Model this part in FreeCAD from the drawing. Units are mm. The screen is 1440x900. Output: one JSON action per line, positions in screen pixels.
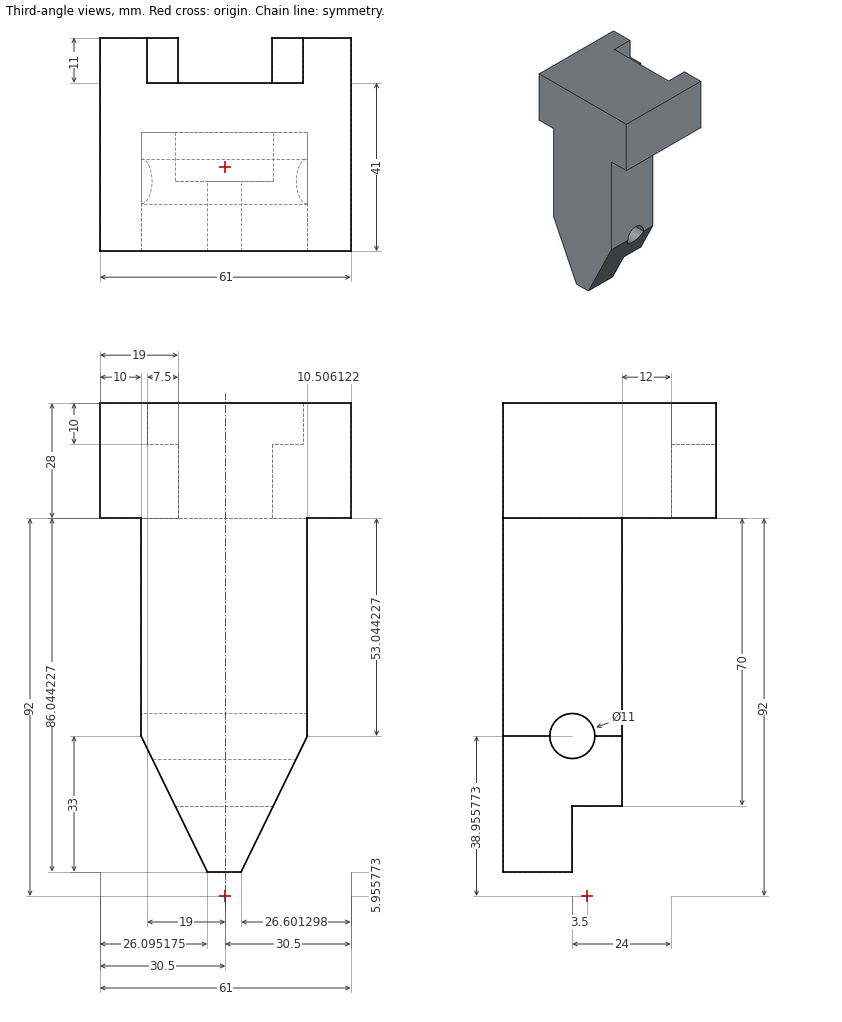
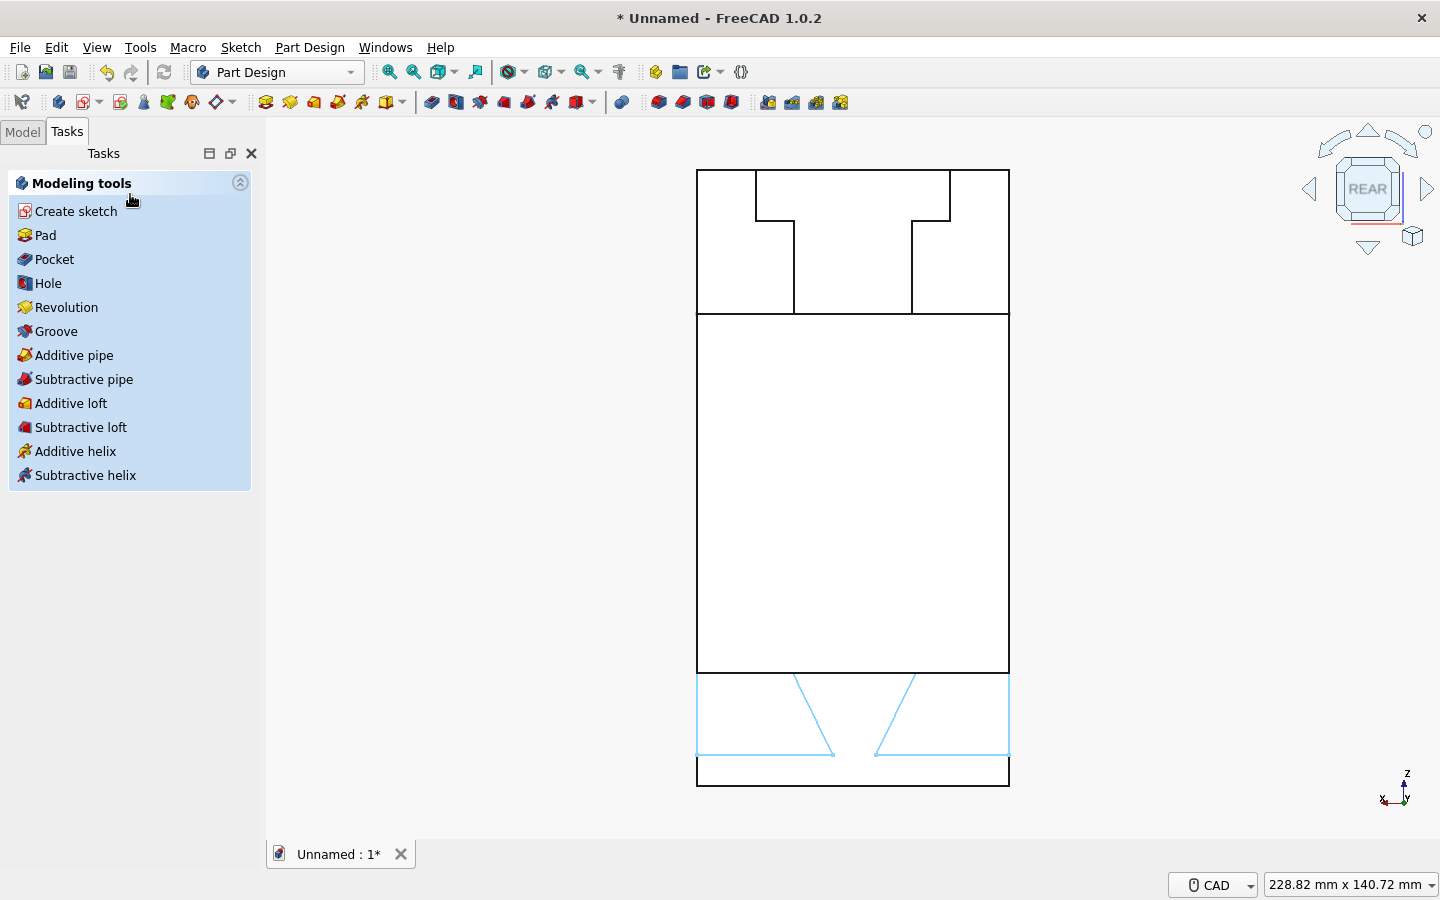
{"action": "left_click", "coordinate": [432, 102]}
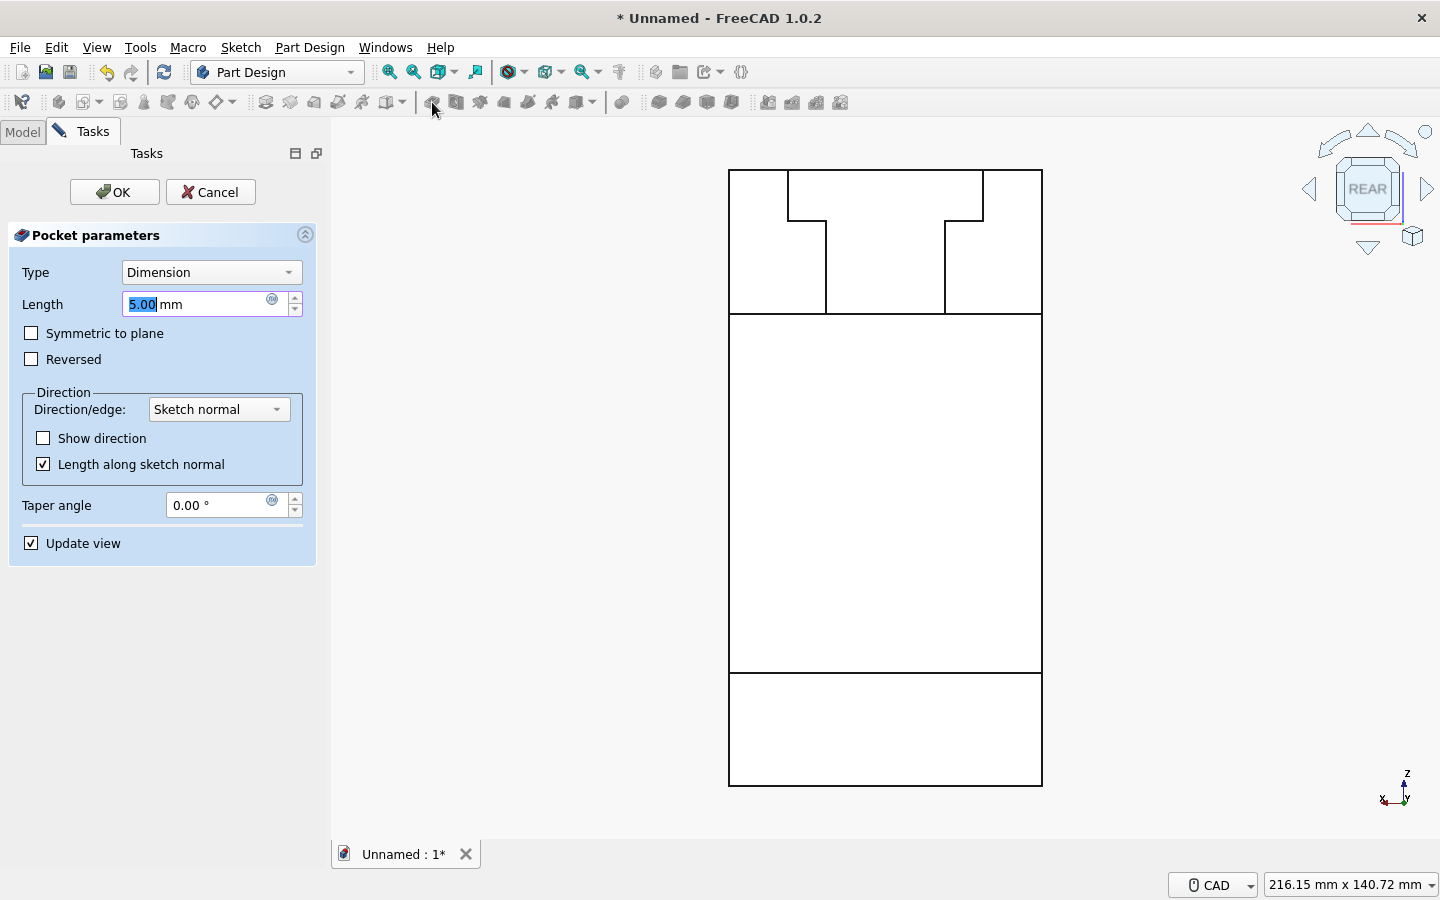
{"action": "left_click", "coordinate": [212, 272]}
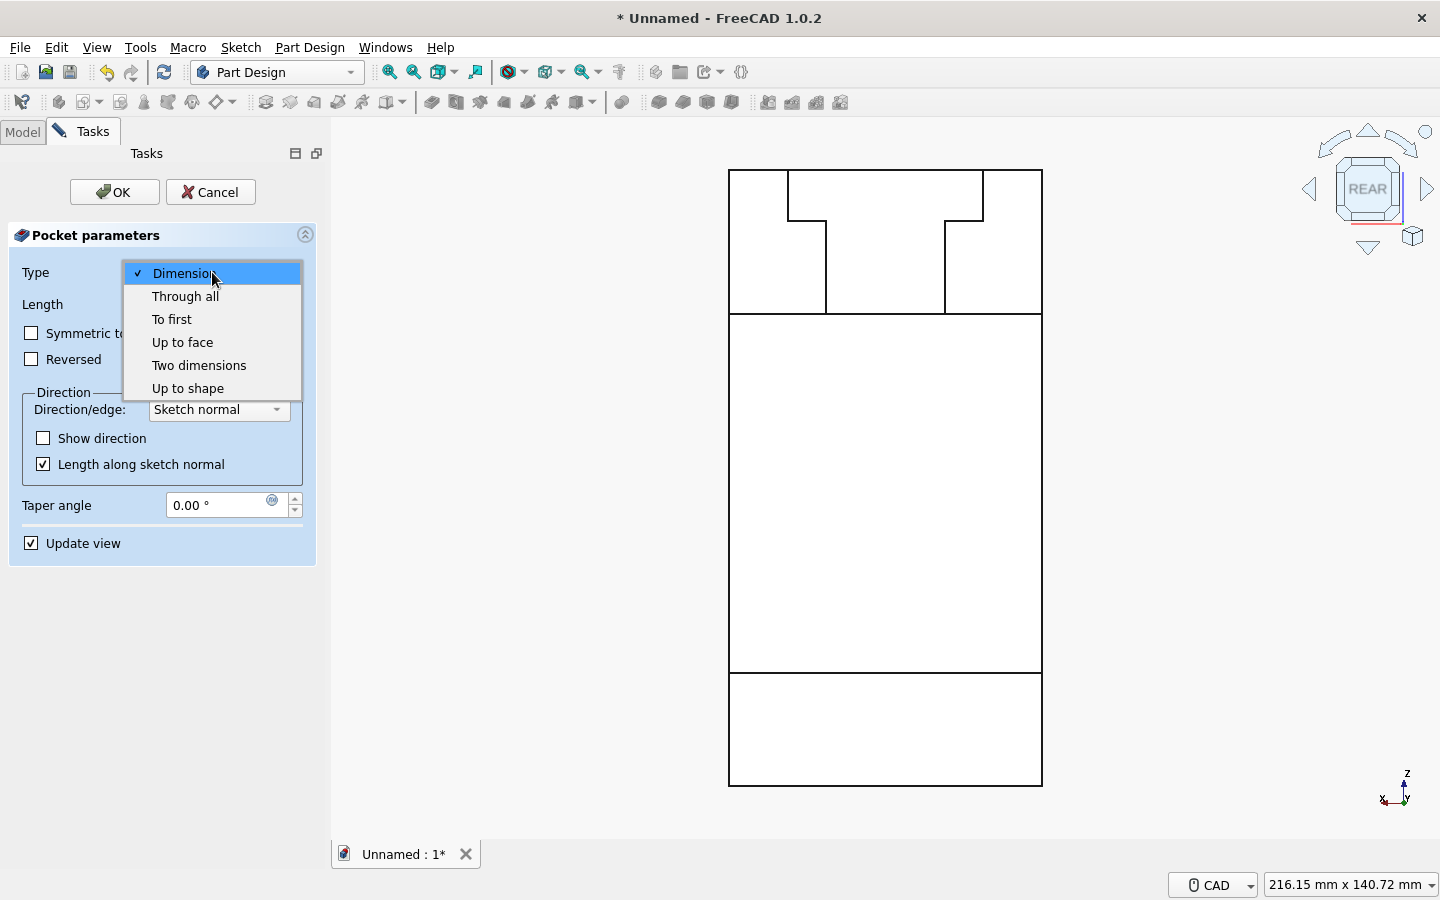
{"action": "left_click", "coordinate": [212, 366]}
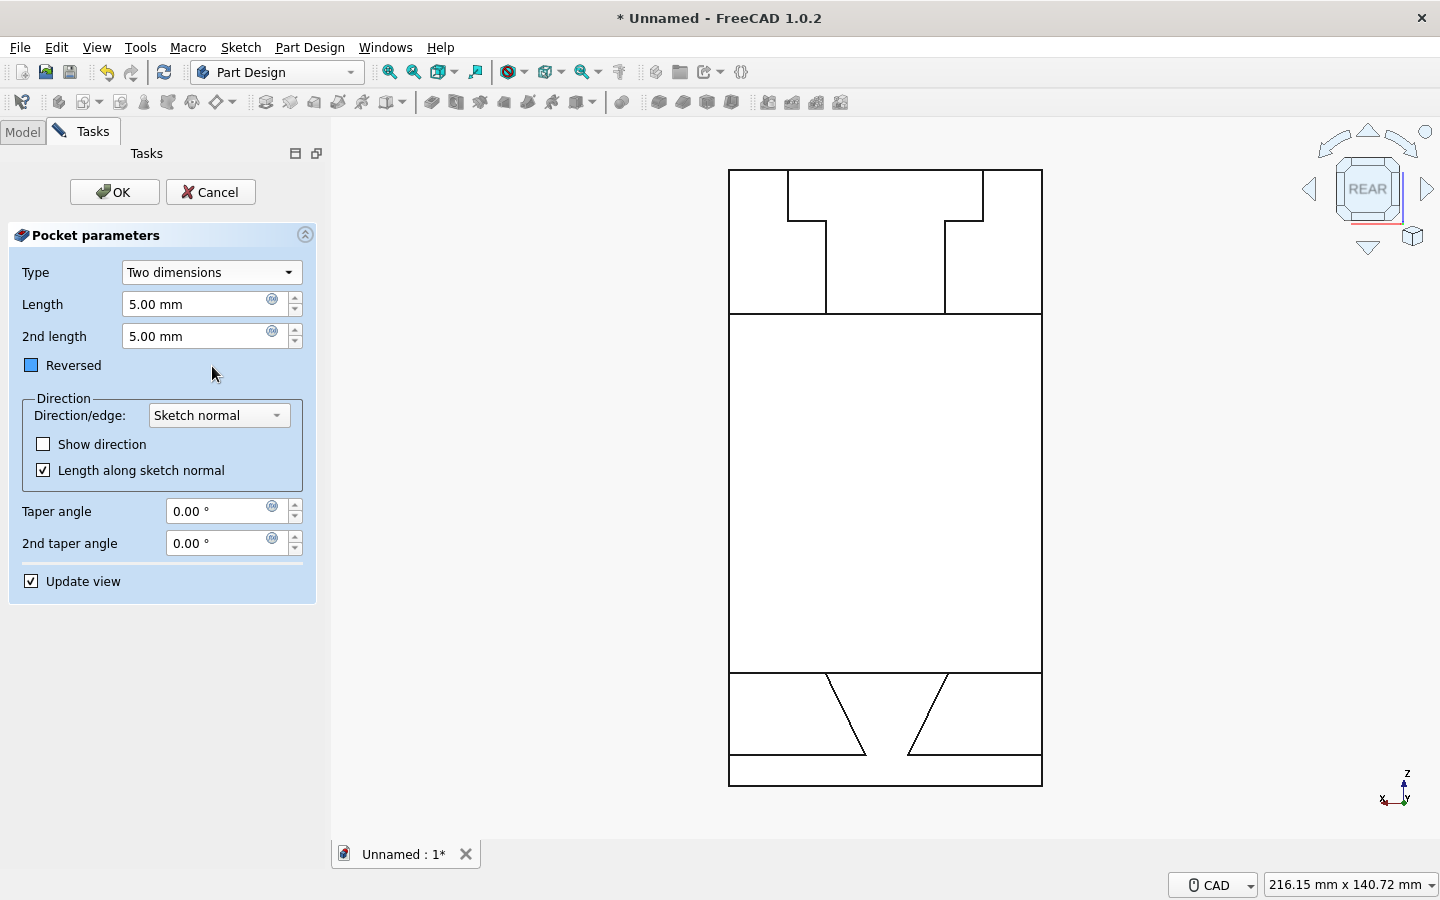
{"action": "triple_click", "coordinate": [204, 304]}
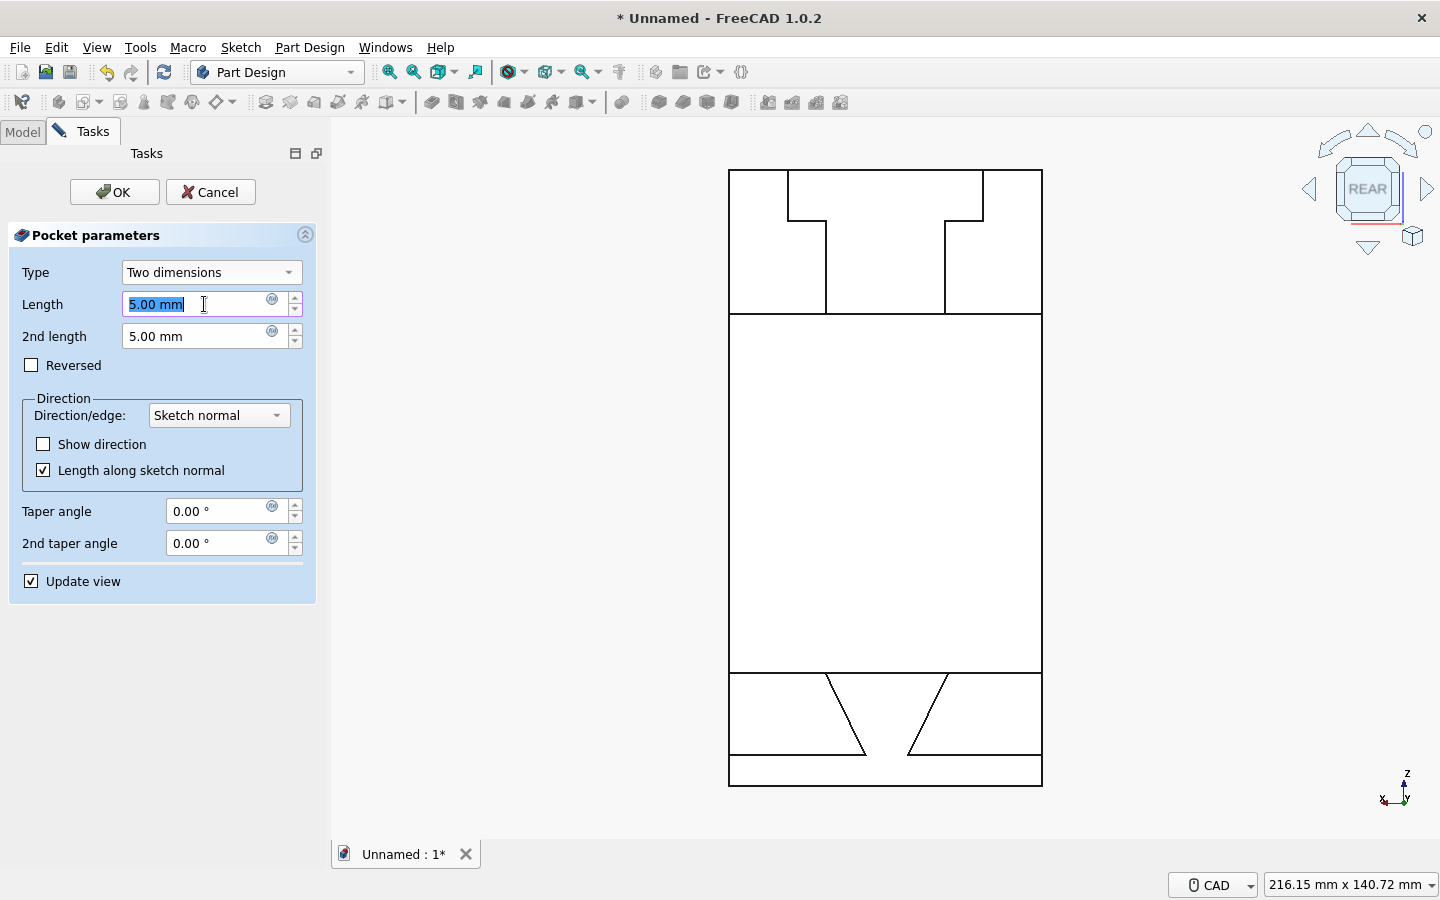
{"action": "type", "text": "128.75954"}
{"action": "key", "text": "Tab"}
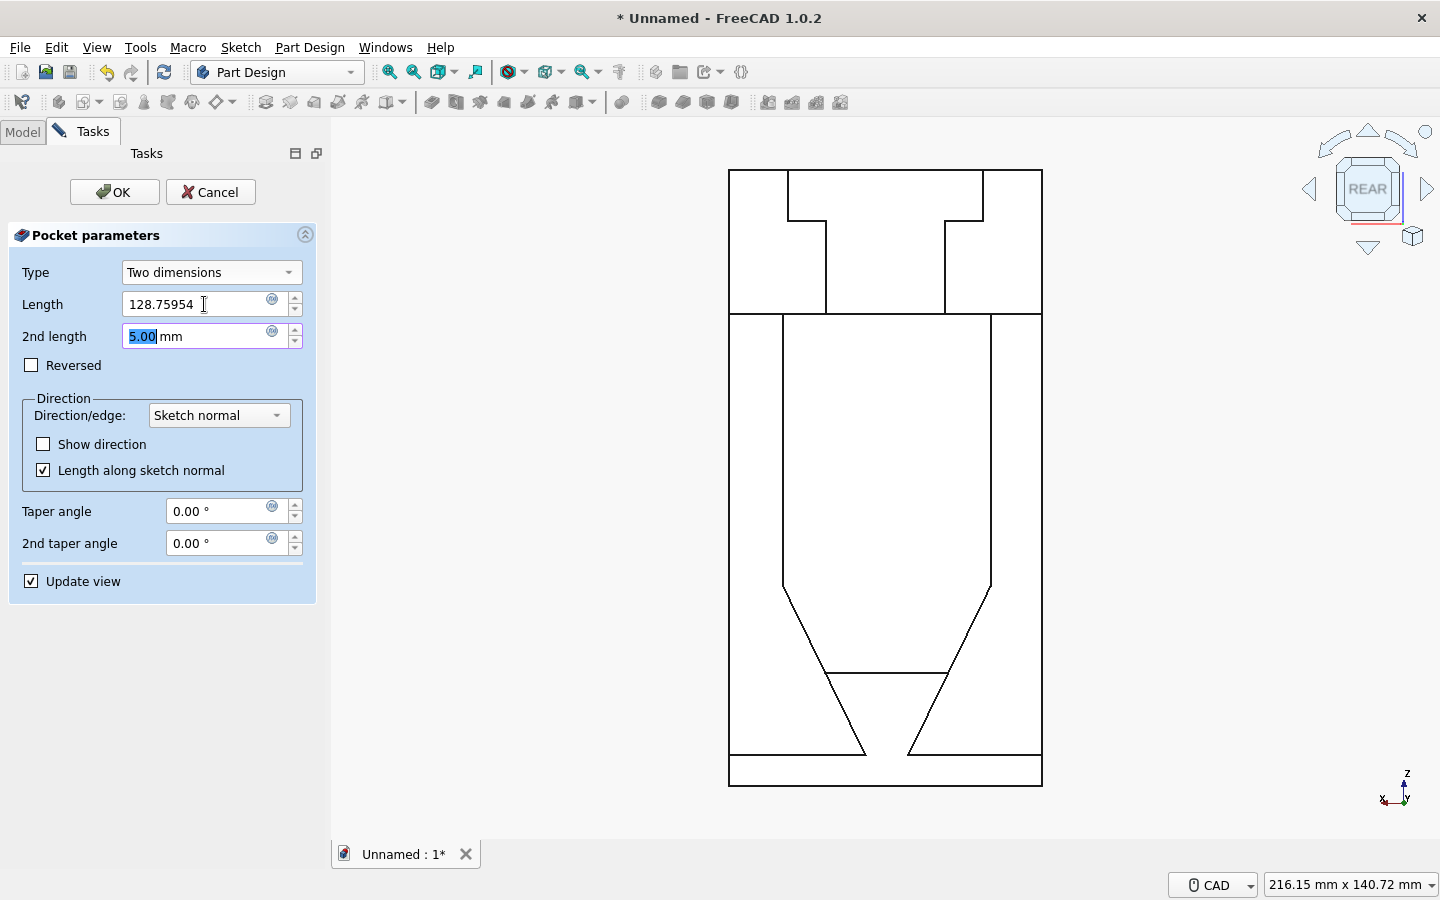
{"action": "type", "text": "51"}
{"action": "key", "text": "Tab"}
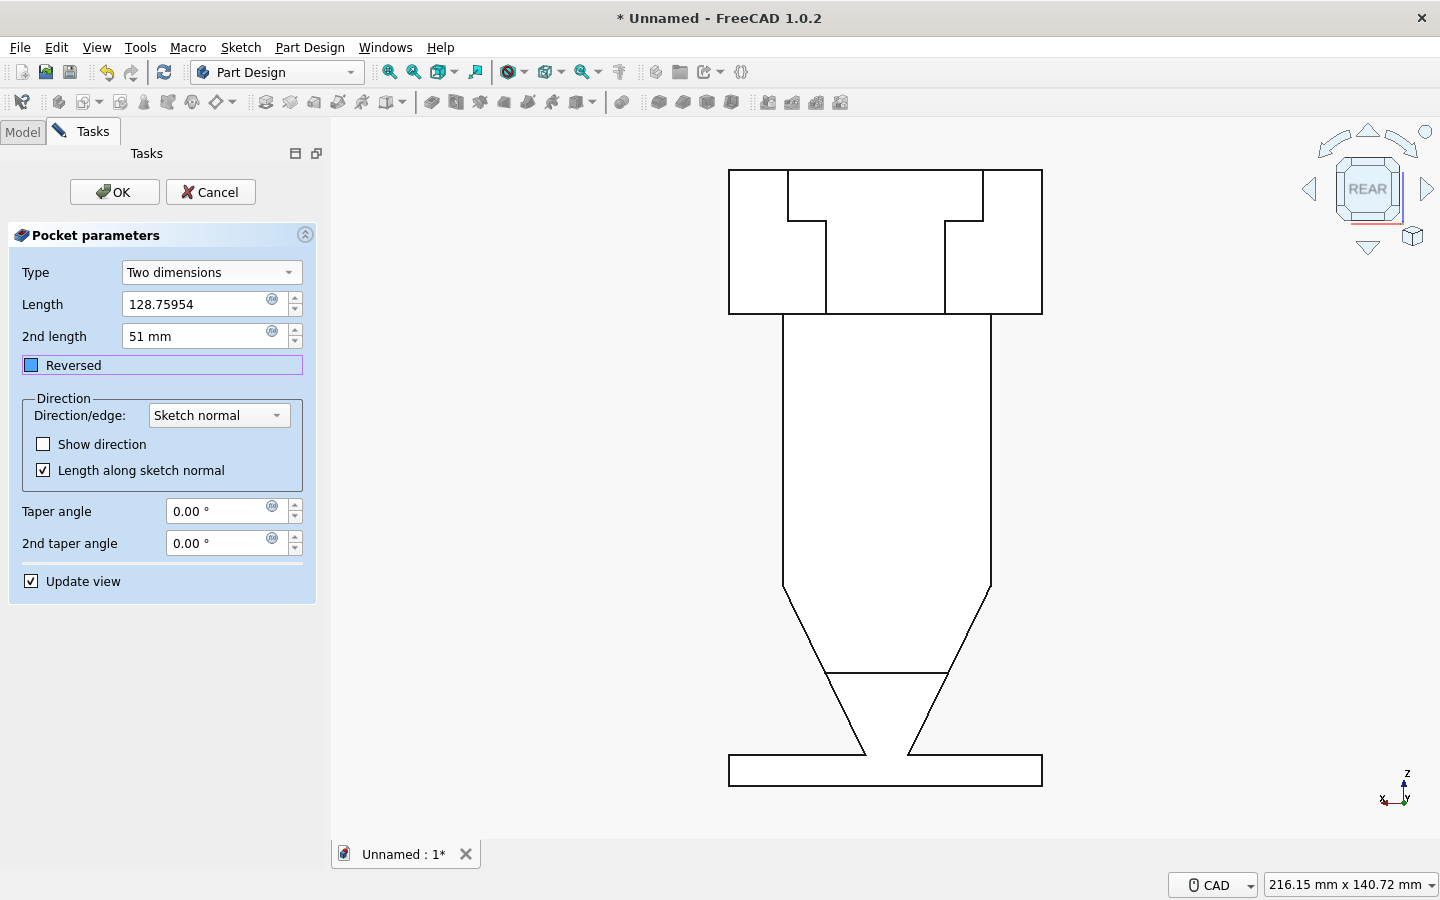
{"action": "left_click", "coordinate": [115, 192]}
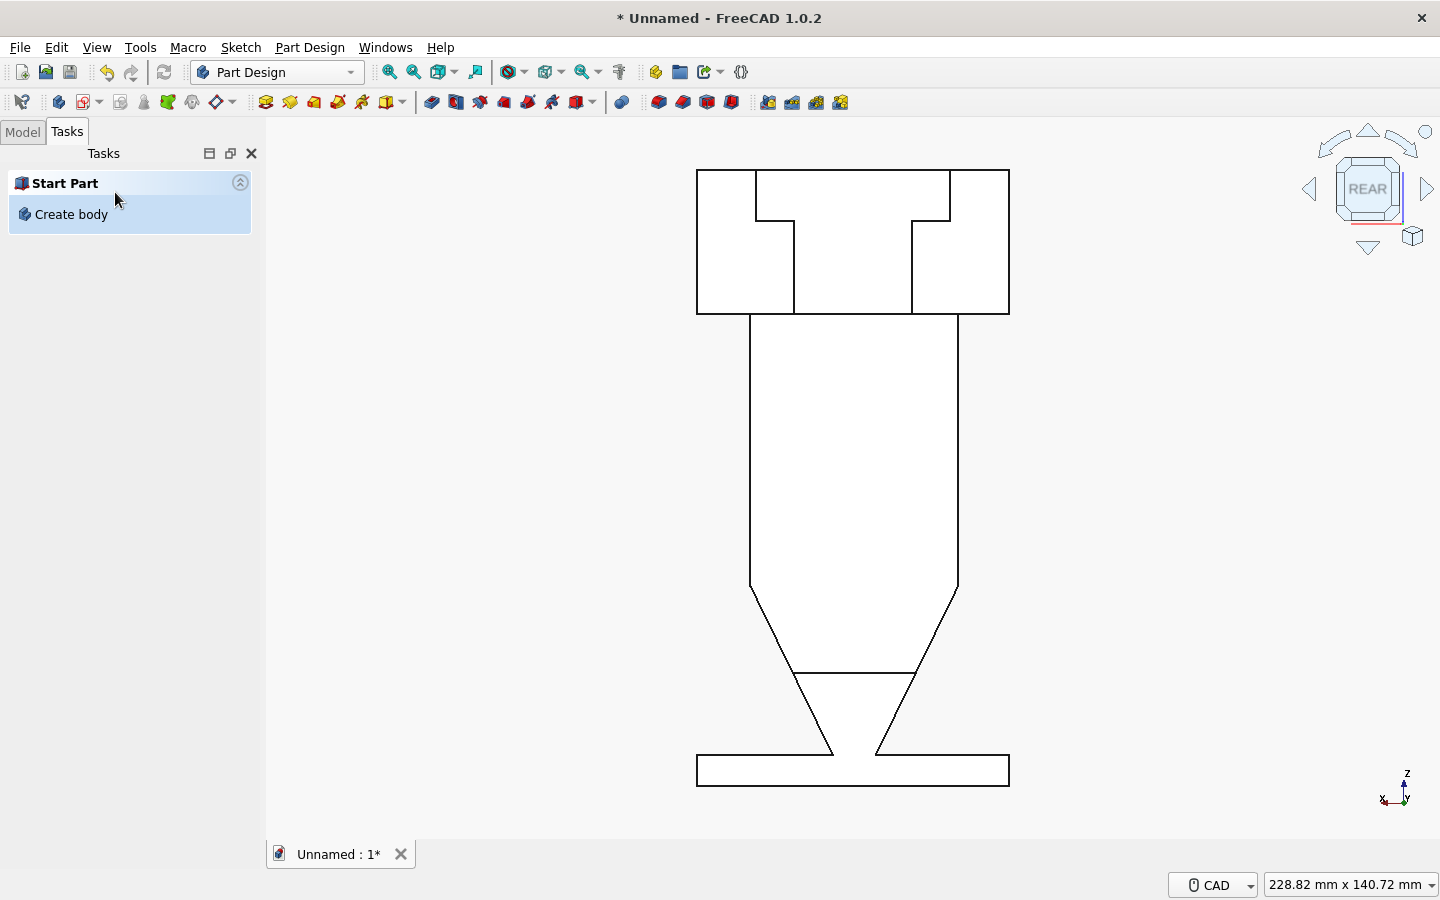
{"action": "left_click", "coordinate": [853, 712]}